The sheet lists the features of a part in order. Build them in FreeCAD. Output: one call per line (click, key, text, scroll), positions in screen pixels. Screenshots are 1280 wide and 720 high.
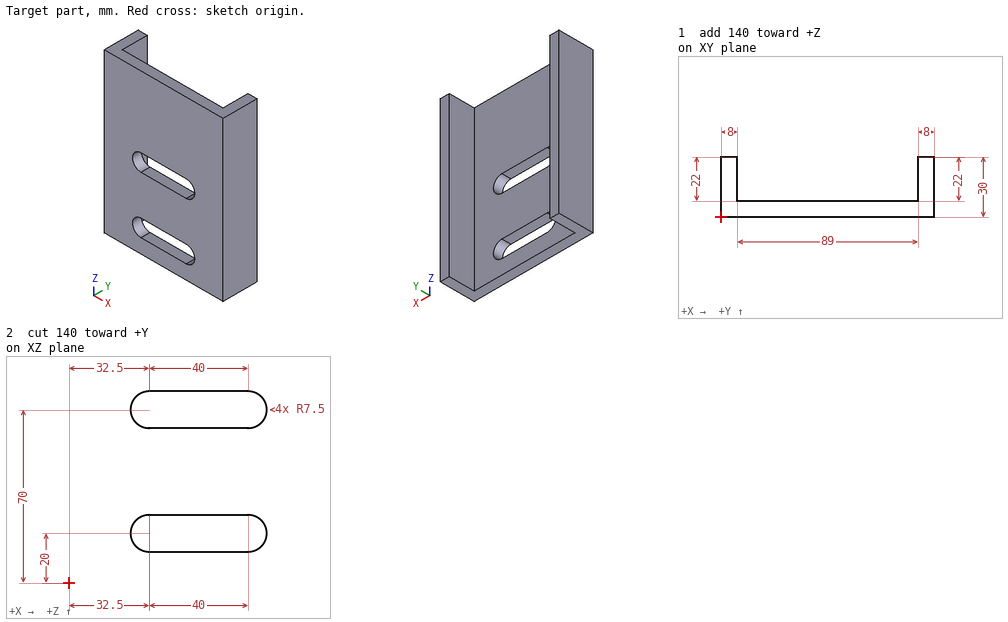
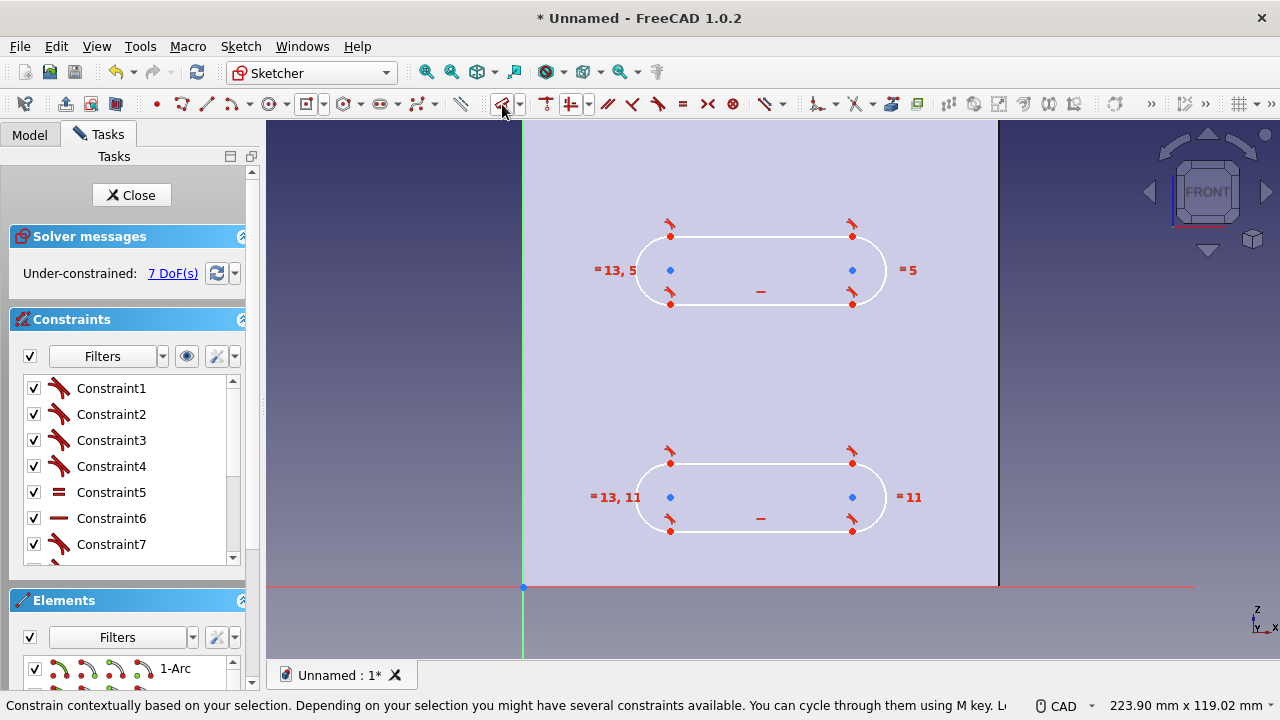
click(642, 251)
click(616, 232)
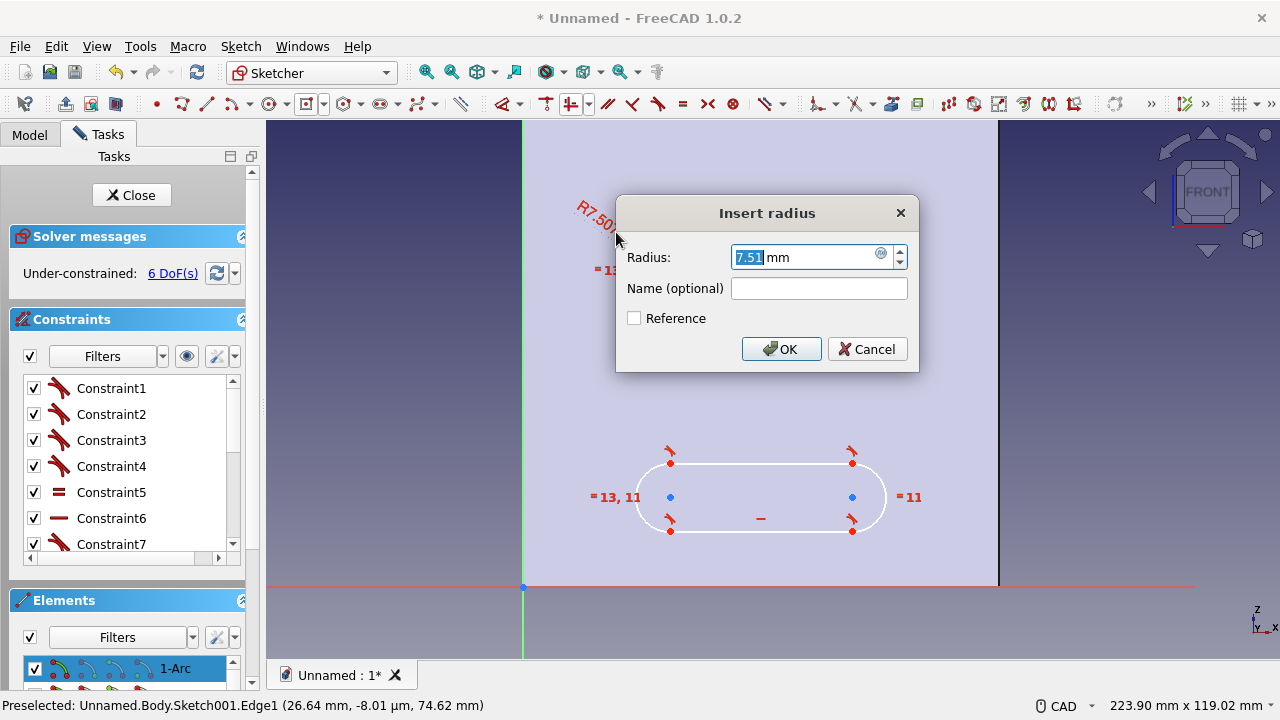
text(7.5)
key(Return)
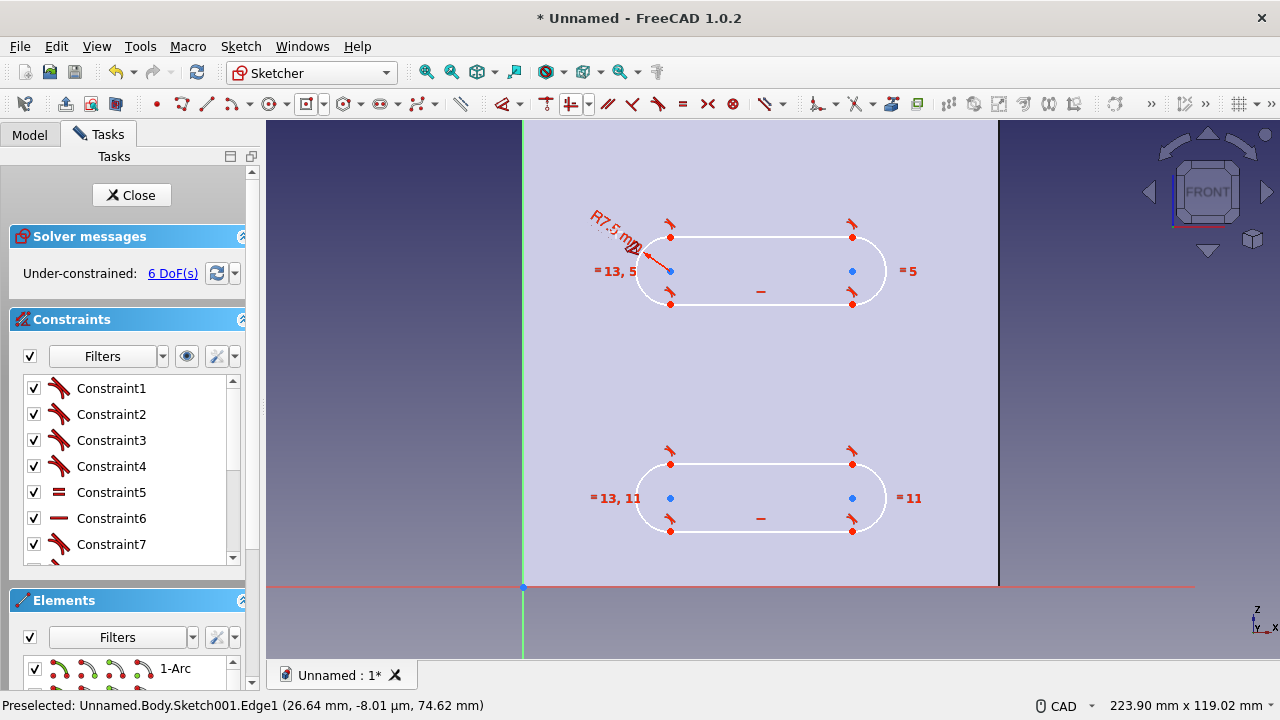
click(725, 237)
click(761, 203)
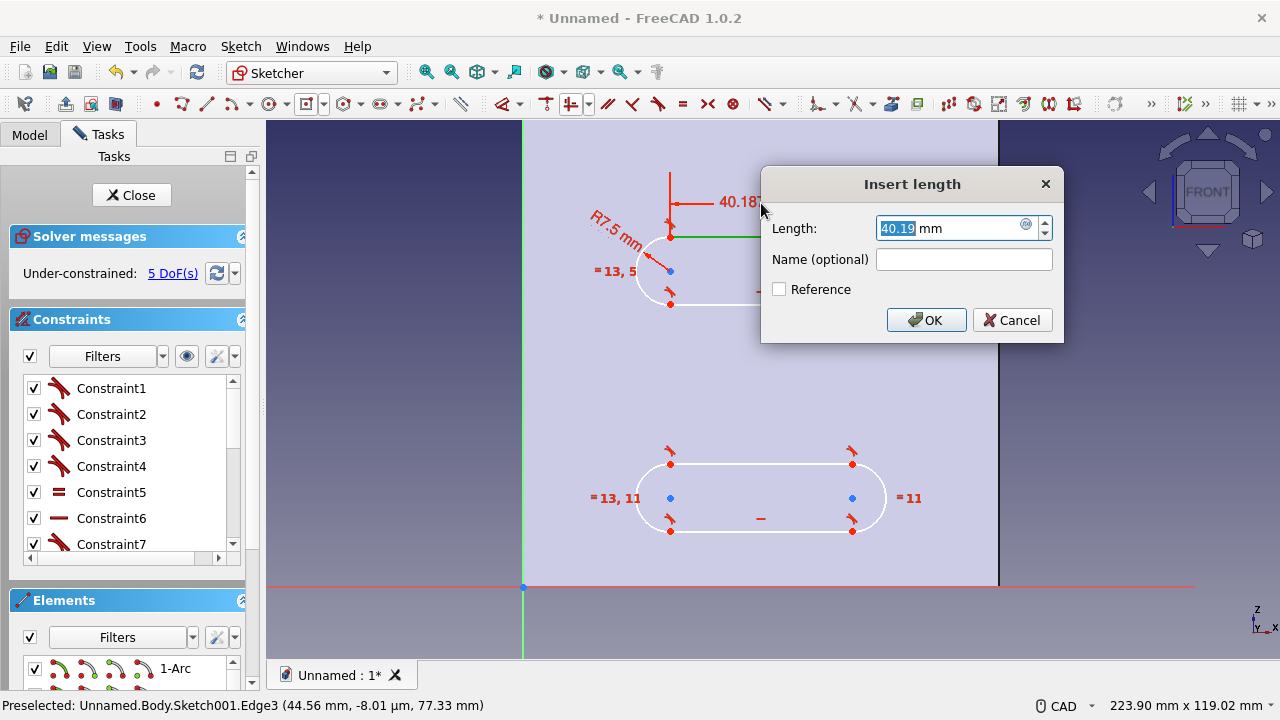
text(40)
key(Return)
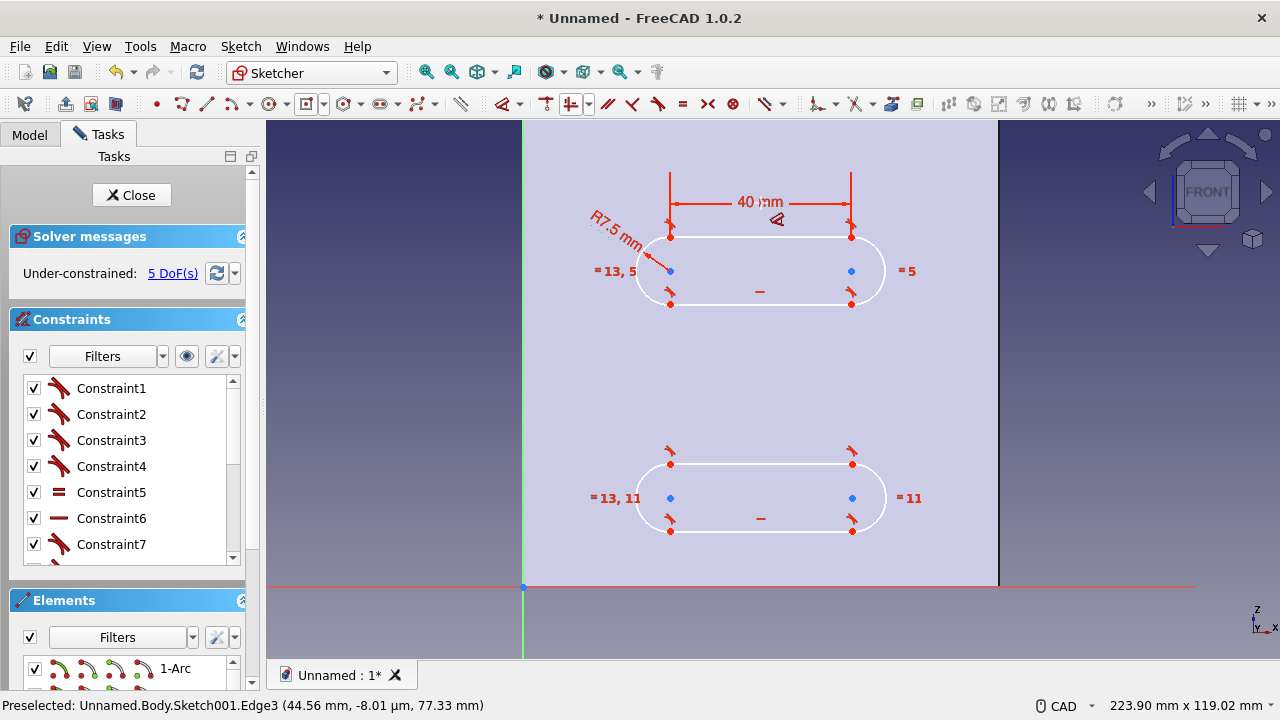
click(725, 464)
click(761, 498)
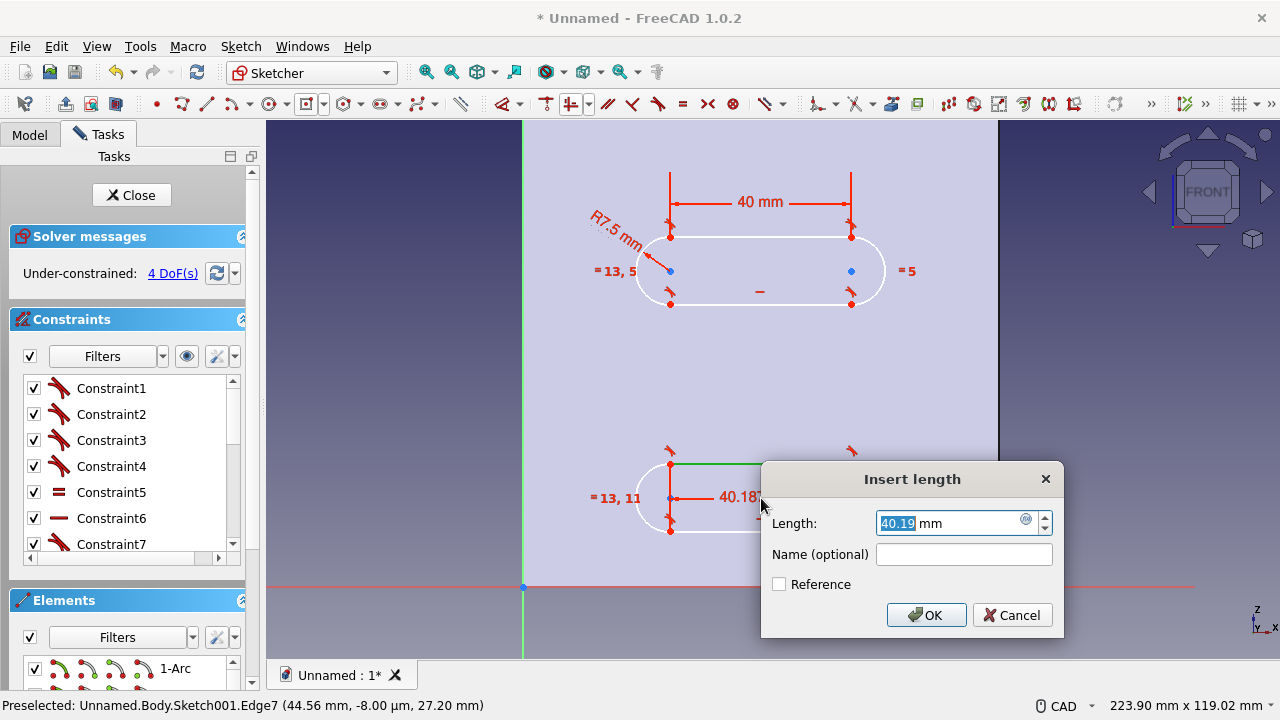
text(40)
key(Return)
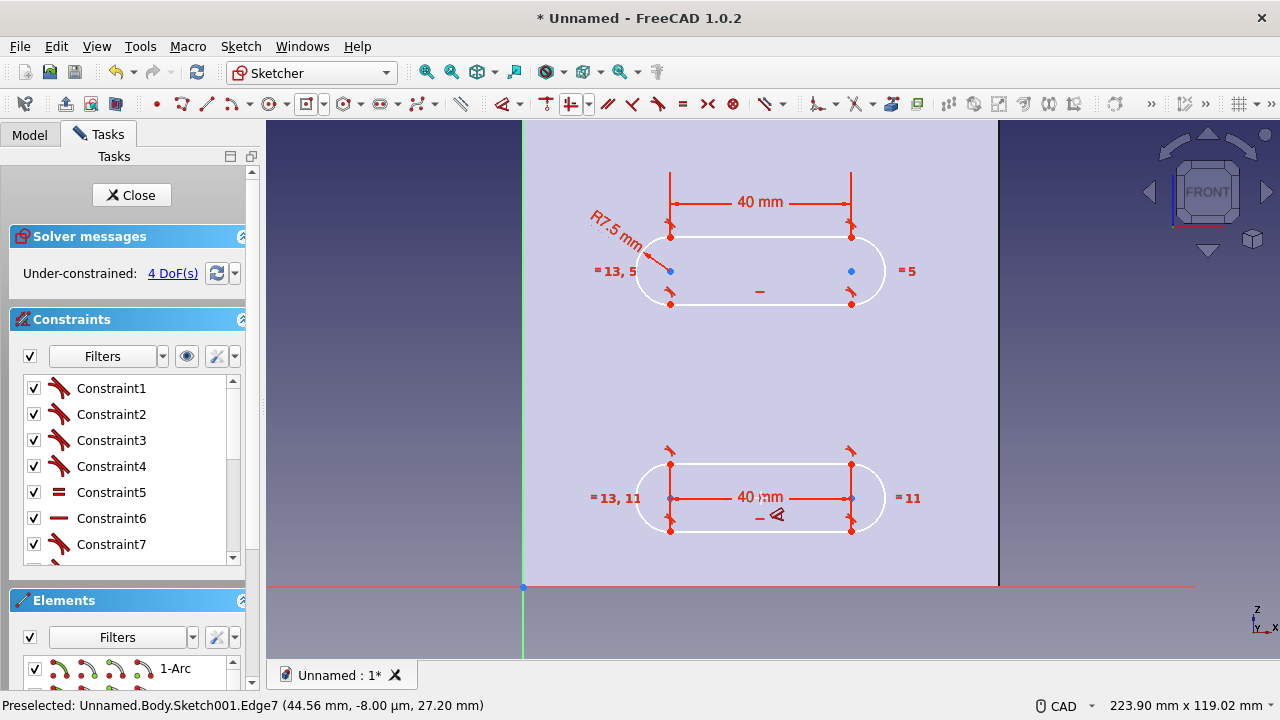
click(670, 271)
click(489, 429)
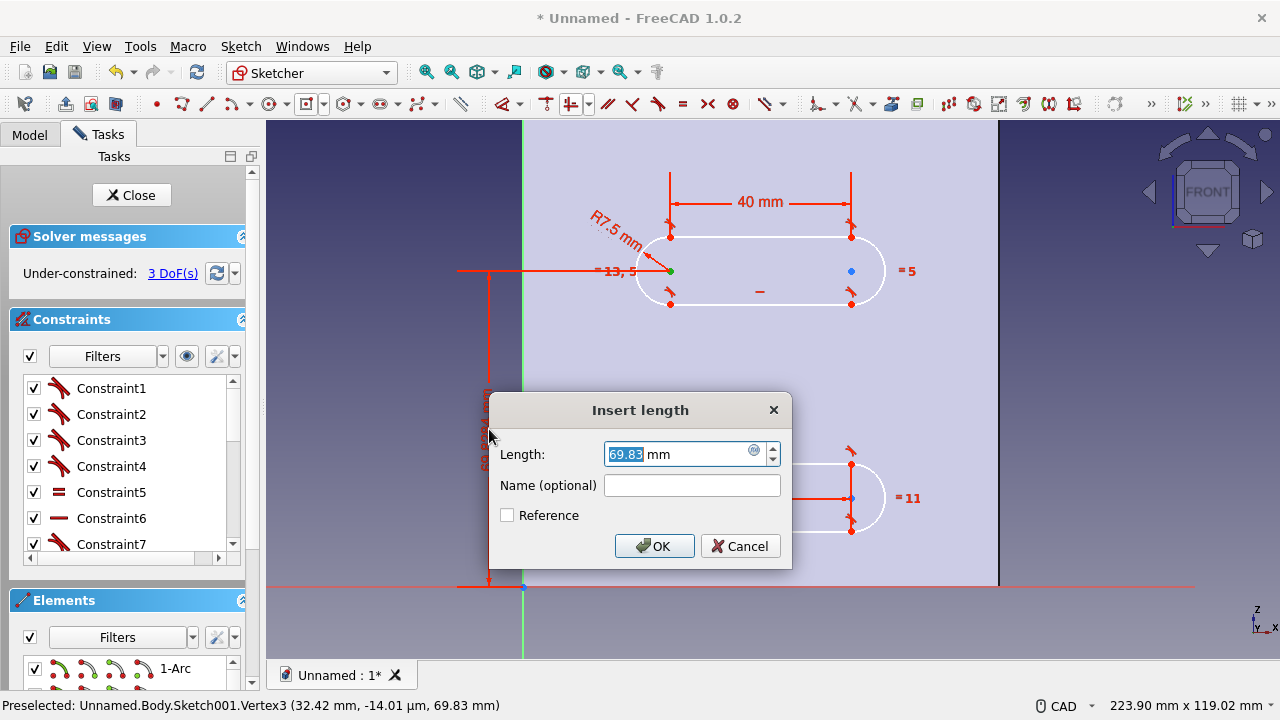
text(70)
key(Return)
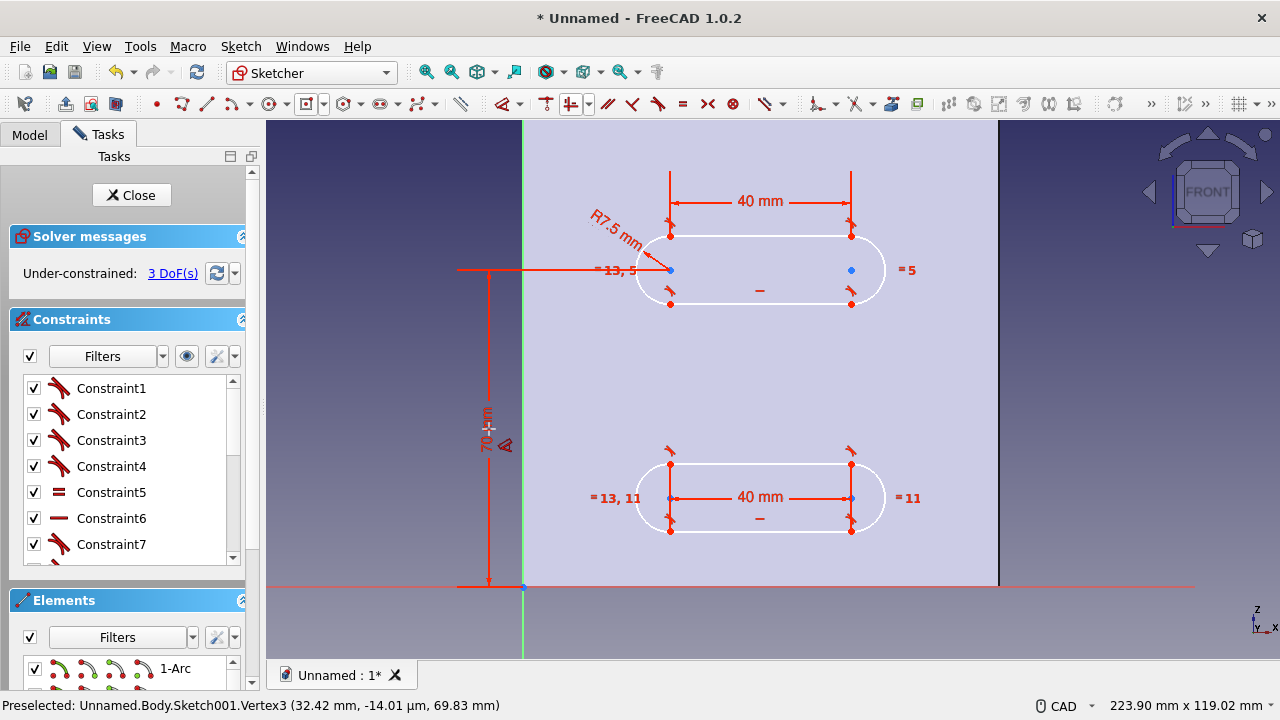
click(670, 498)
click(489, 543)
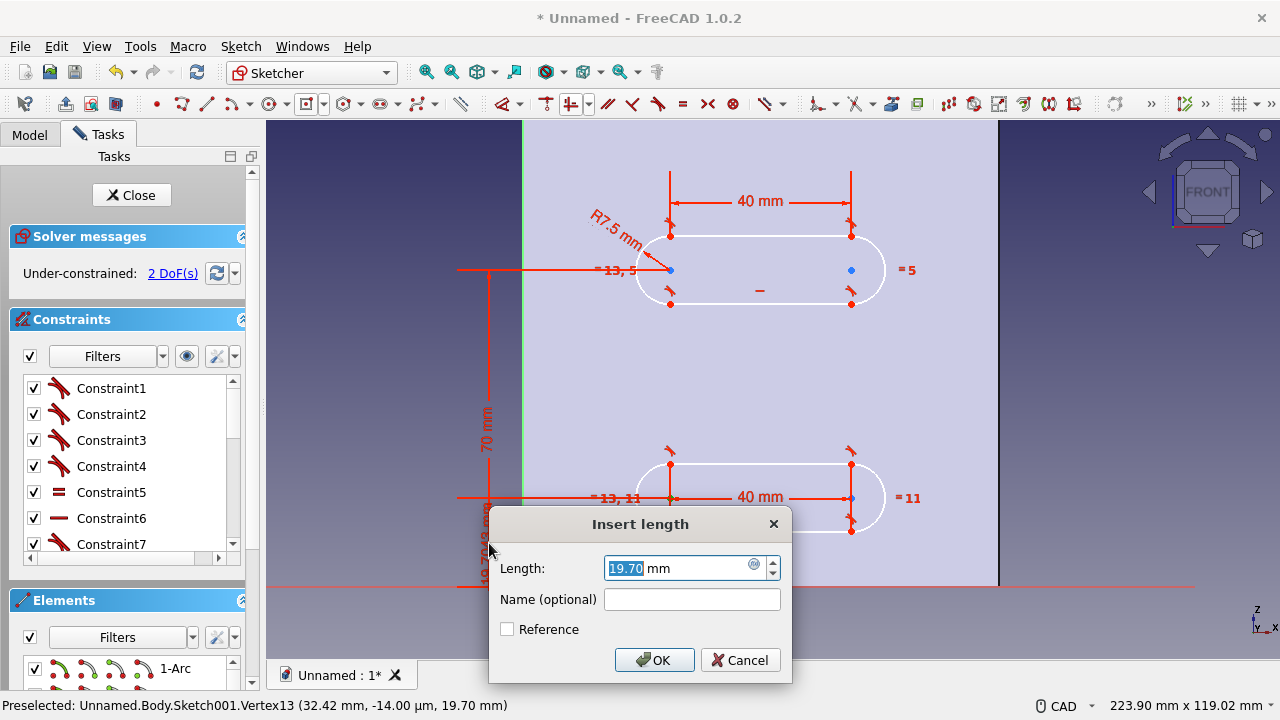
text(20)
key(Return)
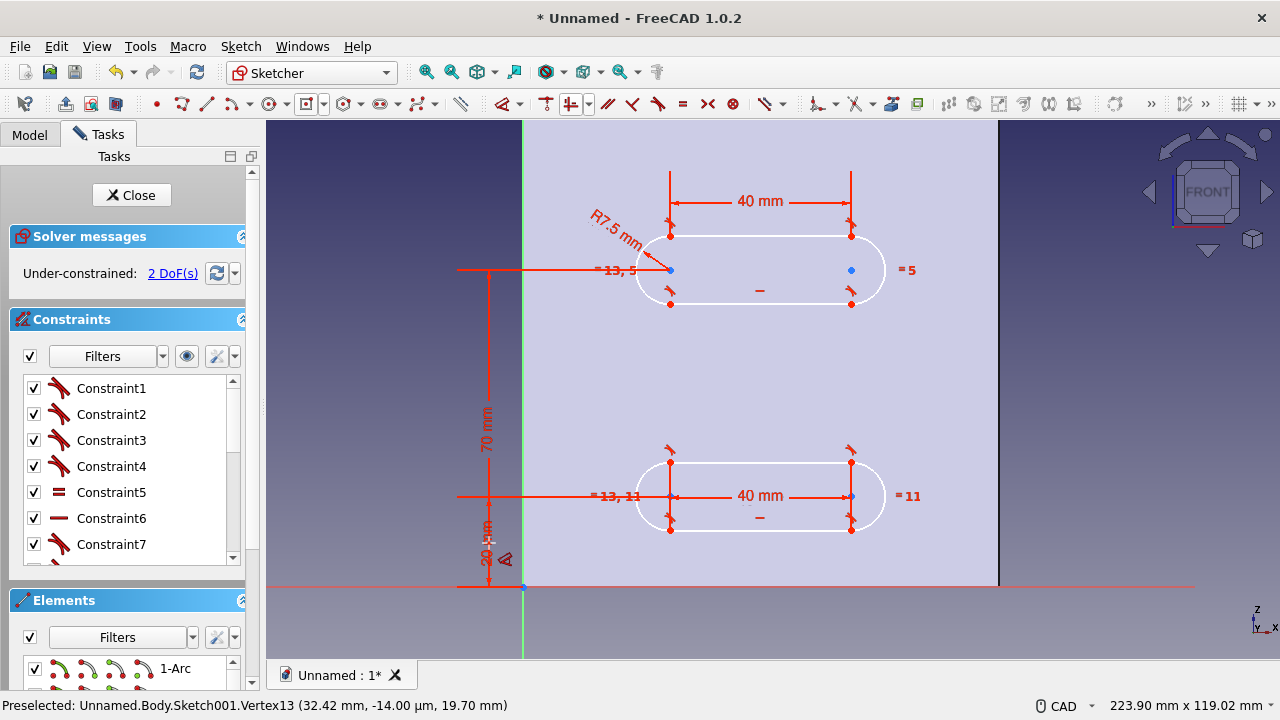
click(670, 236)
click(597, 621)